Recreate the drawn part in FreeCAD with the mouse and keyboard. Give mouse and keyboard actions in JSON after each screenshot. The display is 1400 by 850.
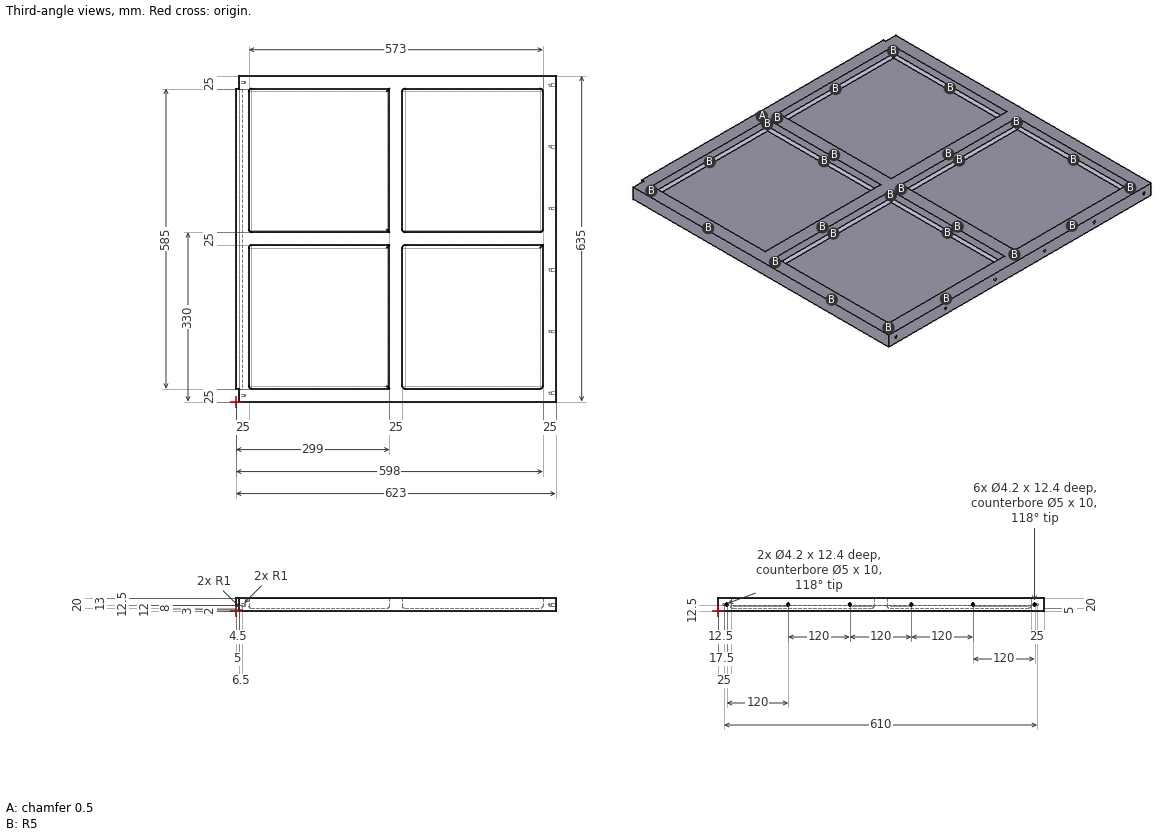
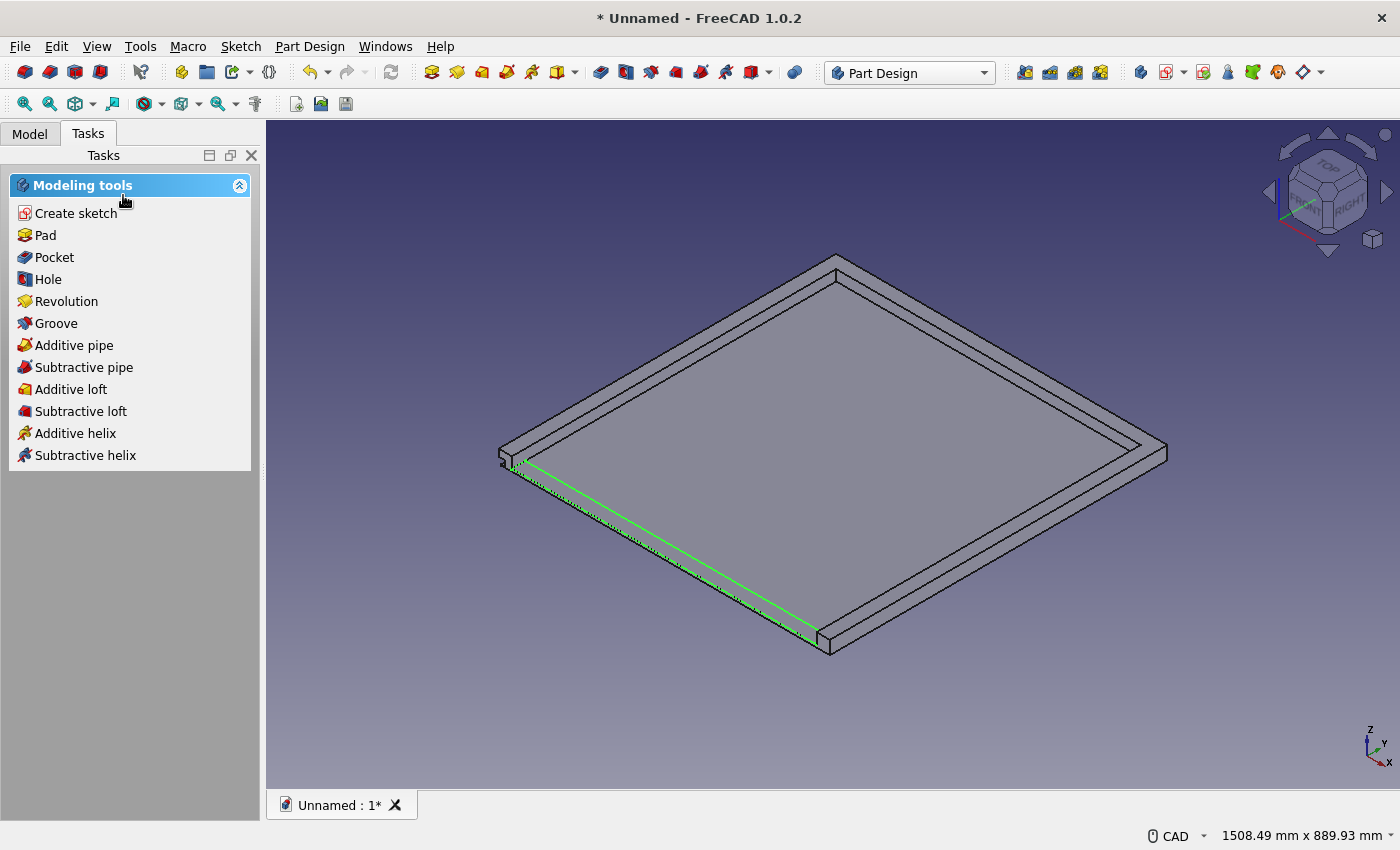
{"action": "left_click", "coordinate": [432, 72]}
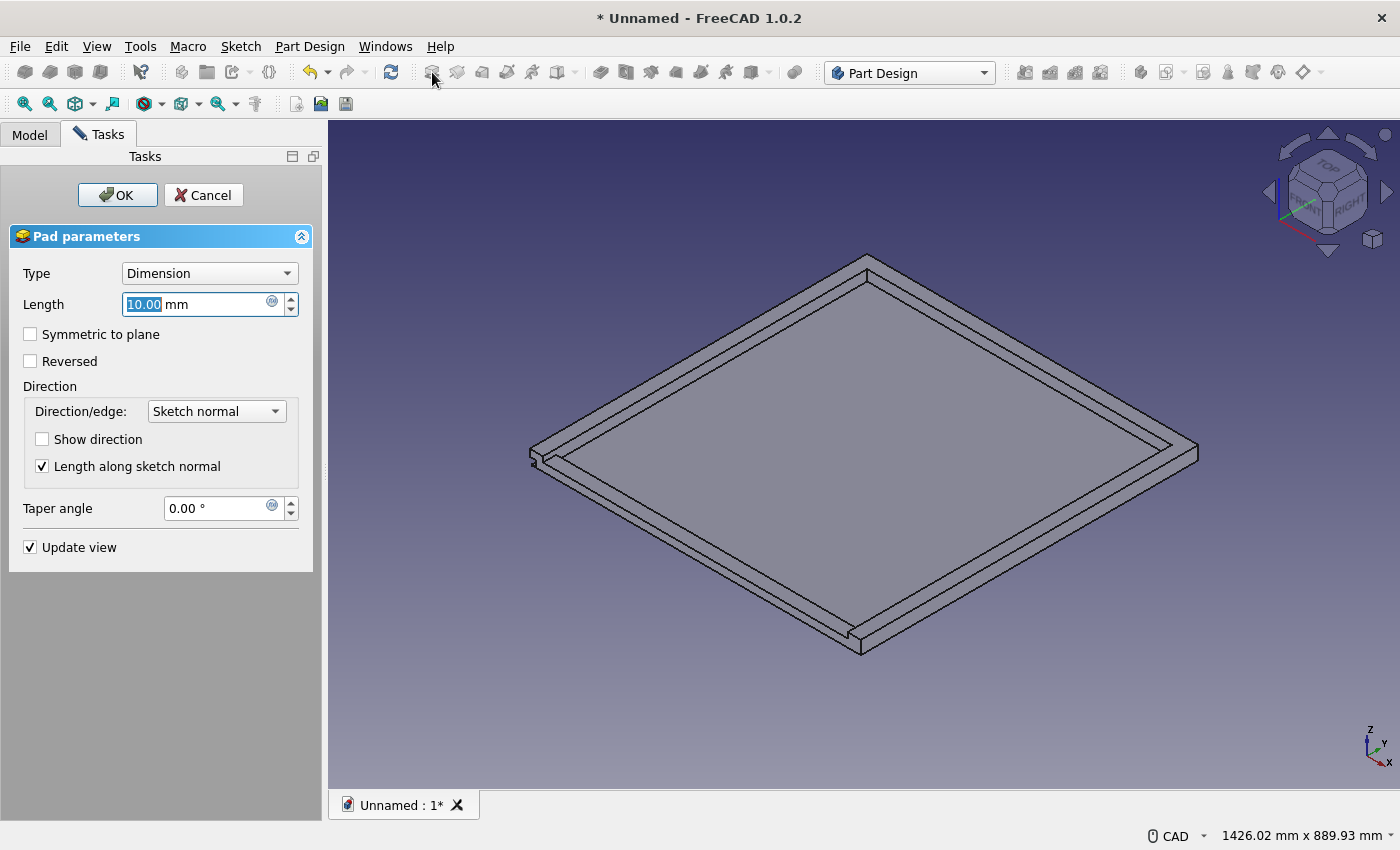
{"action": "type", "text": "20"}
{"action": "key", "text": "Tab"}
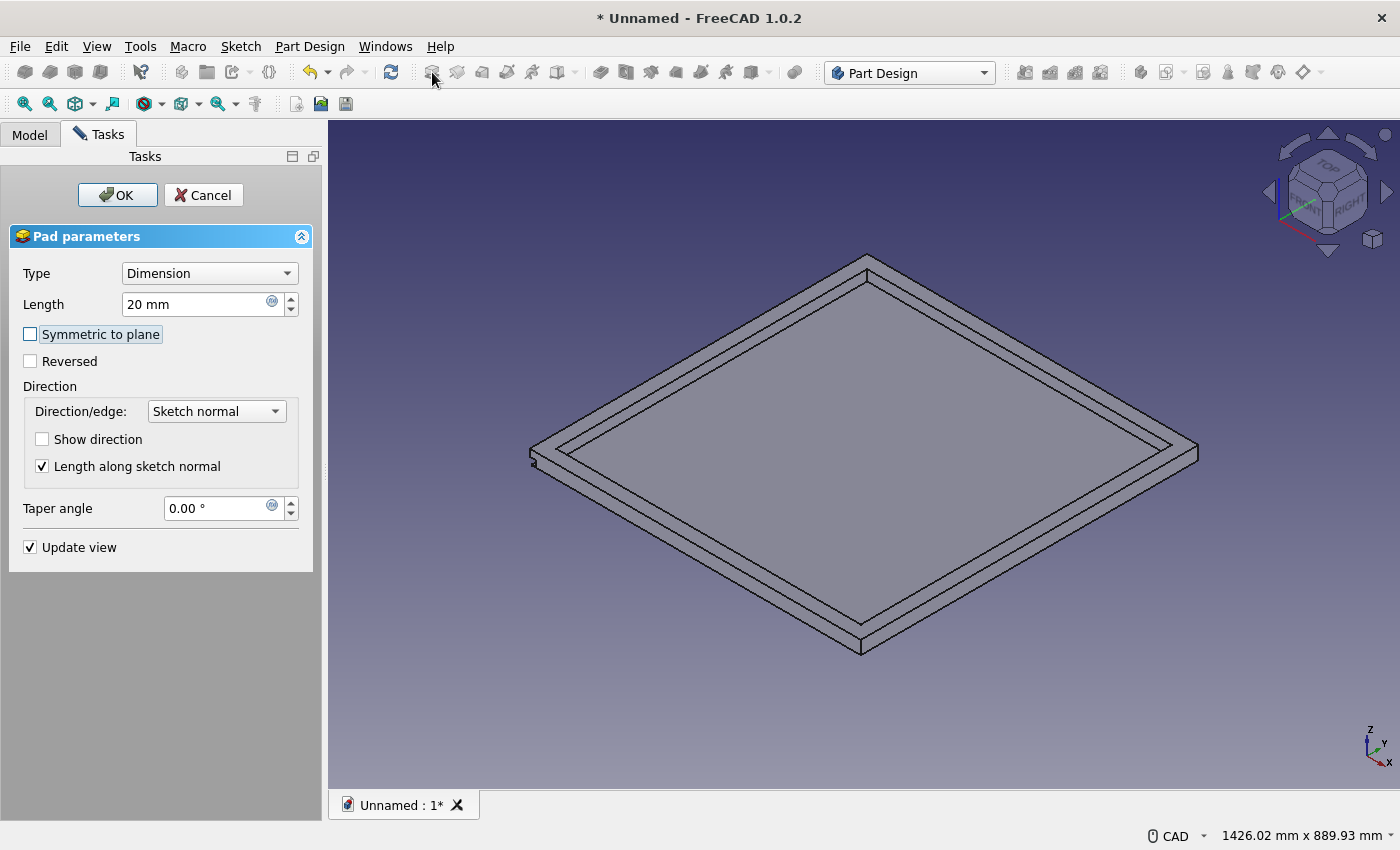
{"action": "left_click", "coordinate": [118, 195]}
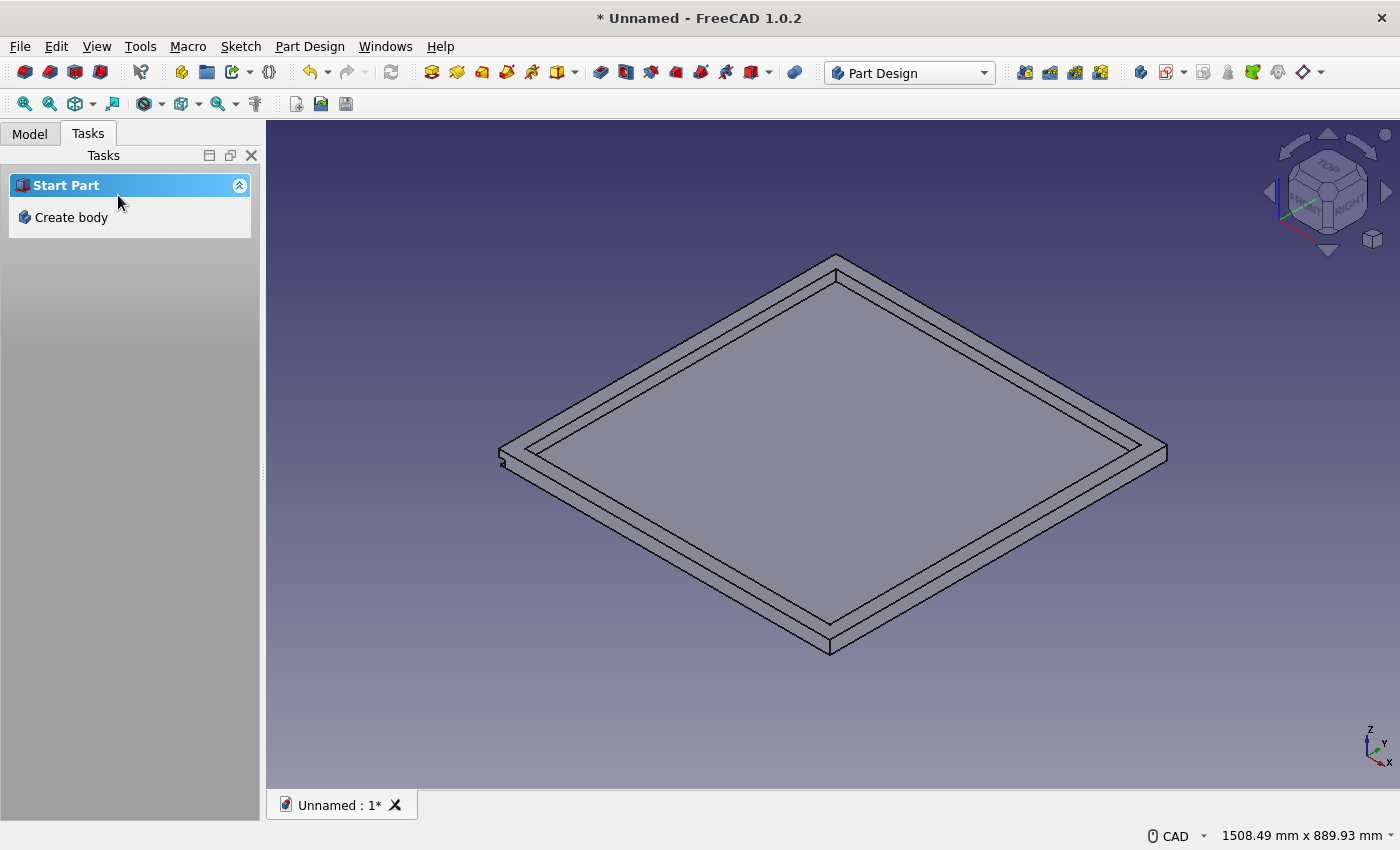
{"action": "left_click", "coordinate": [833, 458]}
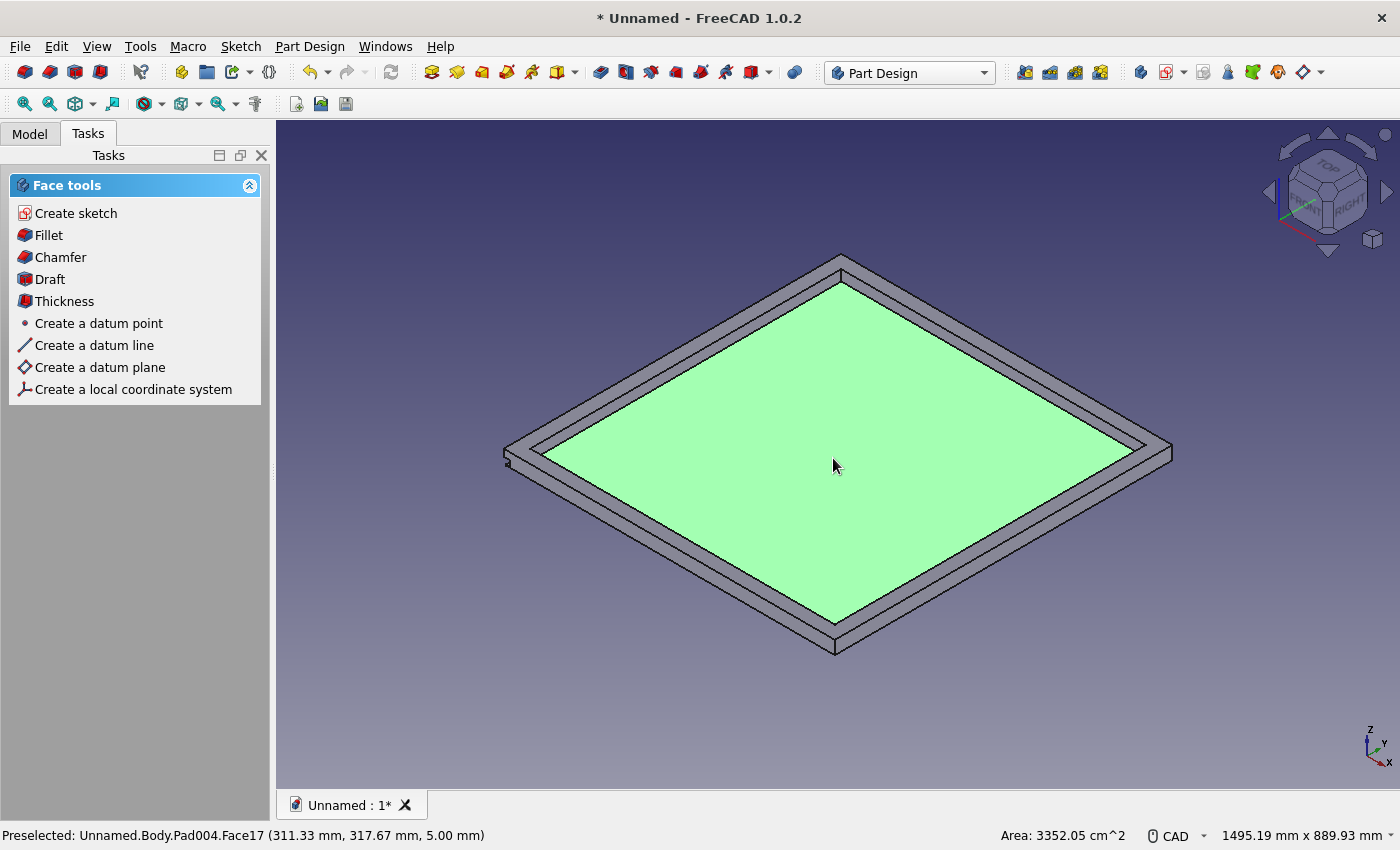
{"action": "left_click", "coordinate": [1166, 72]}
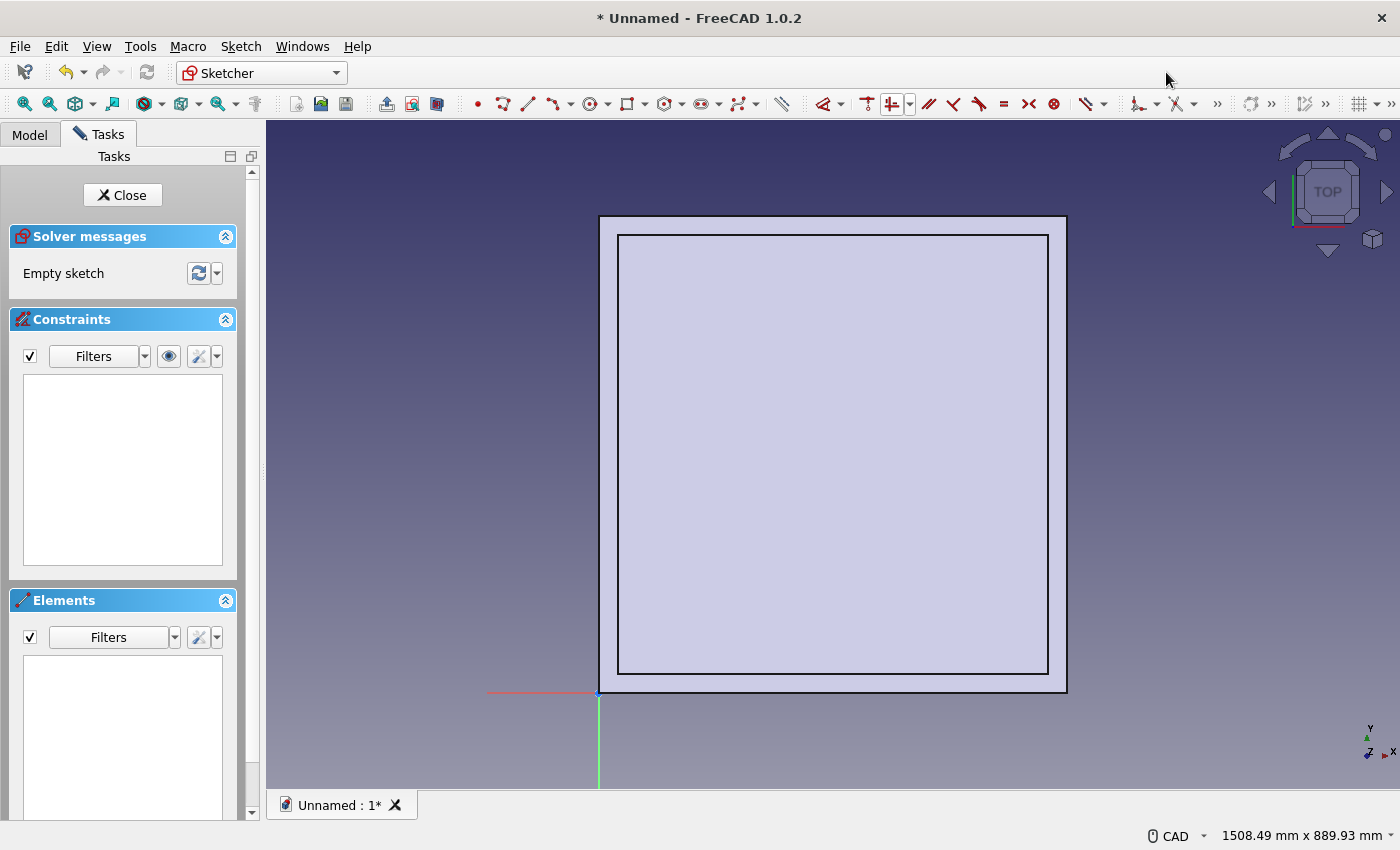
{"action": "scroll", "coordinate": [944, 761], "scroll_direction": "up", "scroll_amount": 2}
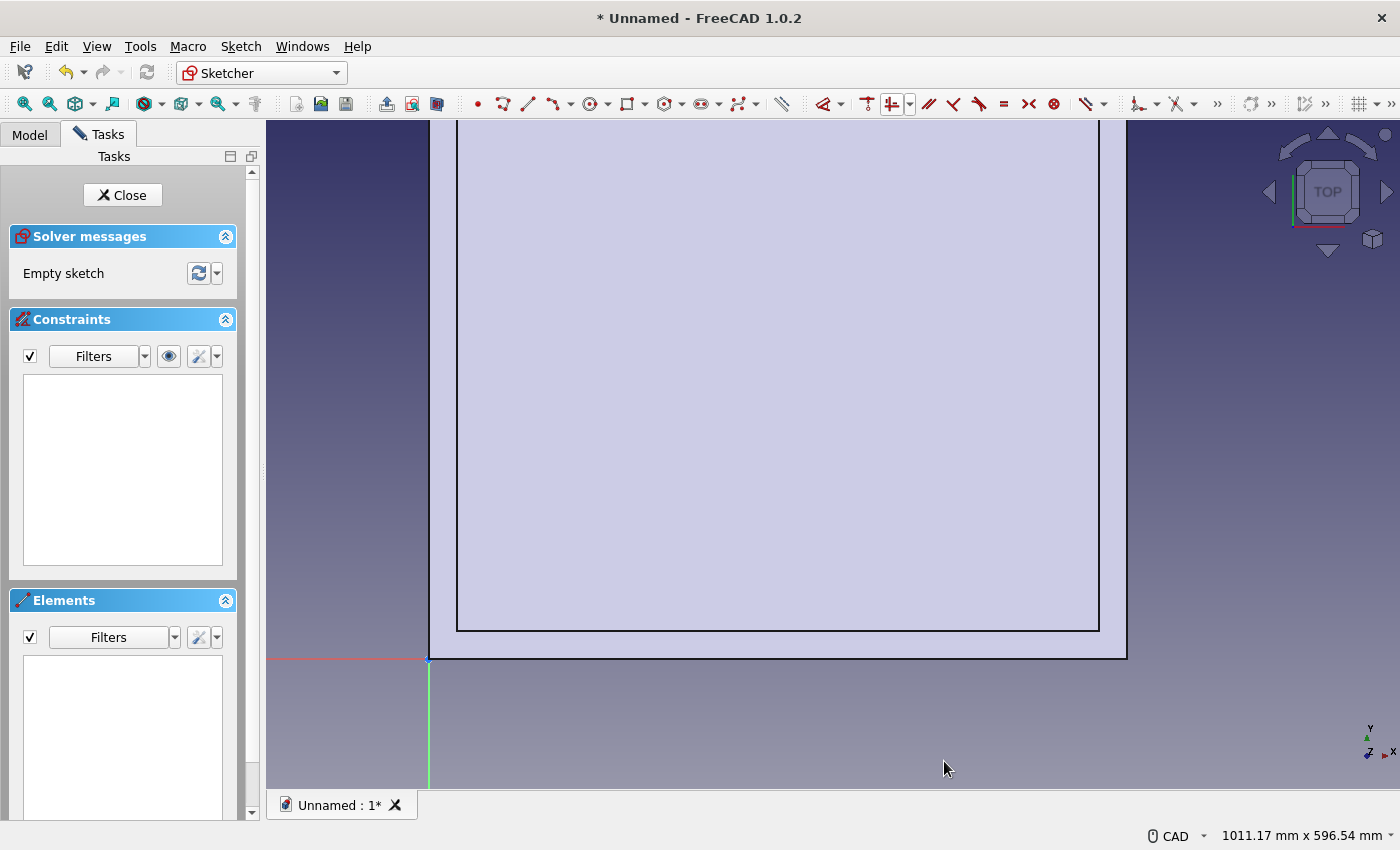
{"action": "left_click", "coordinate": [626, 104]}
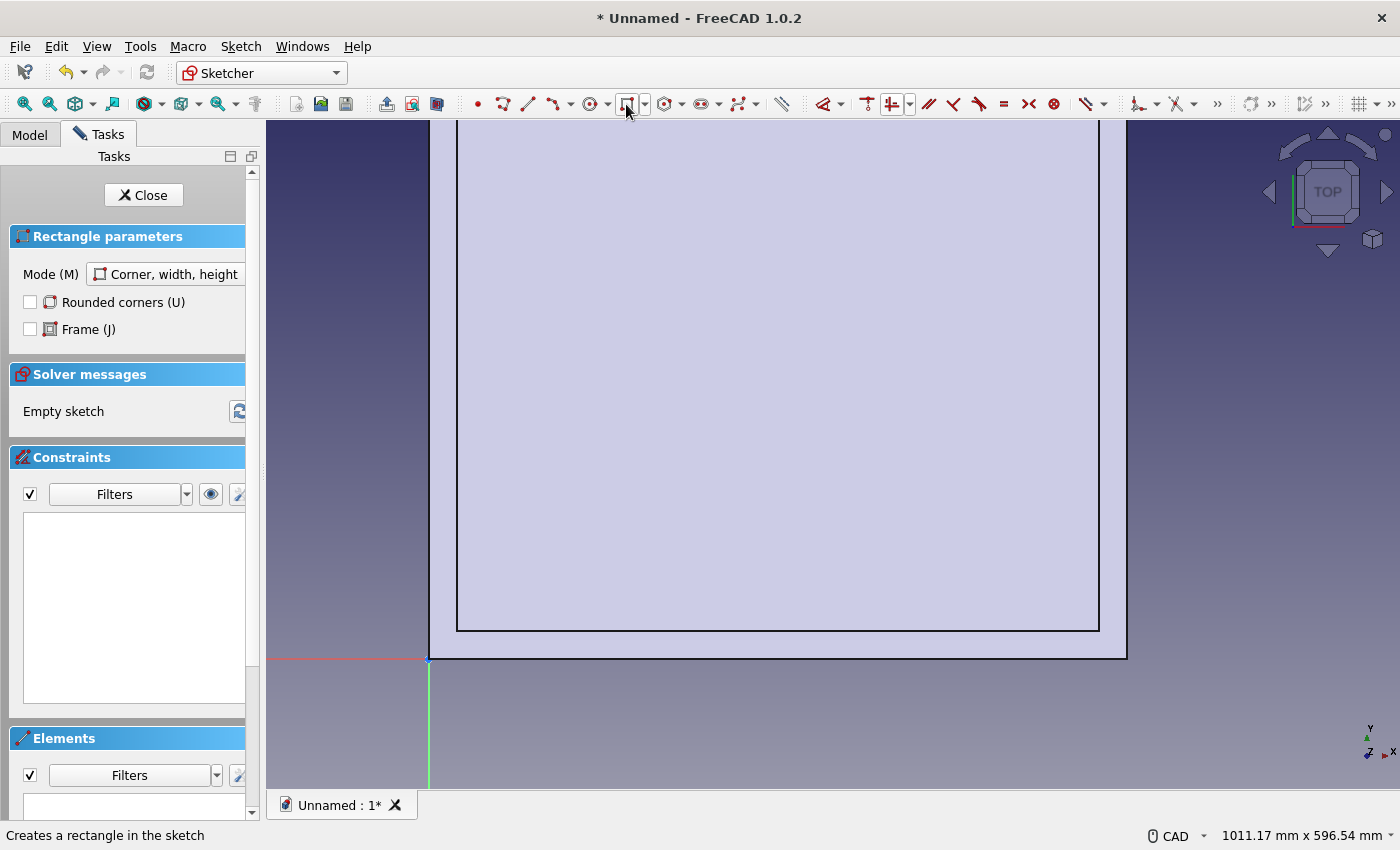
{"action": "left_click", "coordinate": [457, 289]}
{"action": "left_click", "coordinate": [1099, 317]}
{"action": "key", "text": "Escape"}